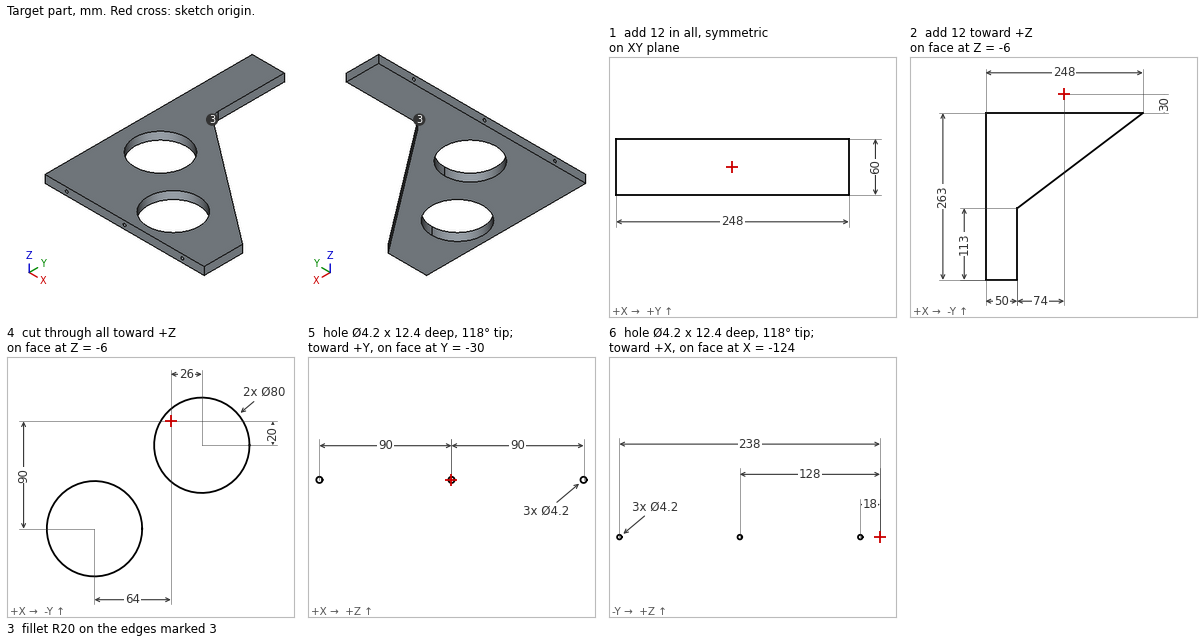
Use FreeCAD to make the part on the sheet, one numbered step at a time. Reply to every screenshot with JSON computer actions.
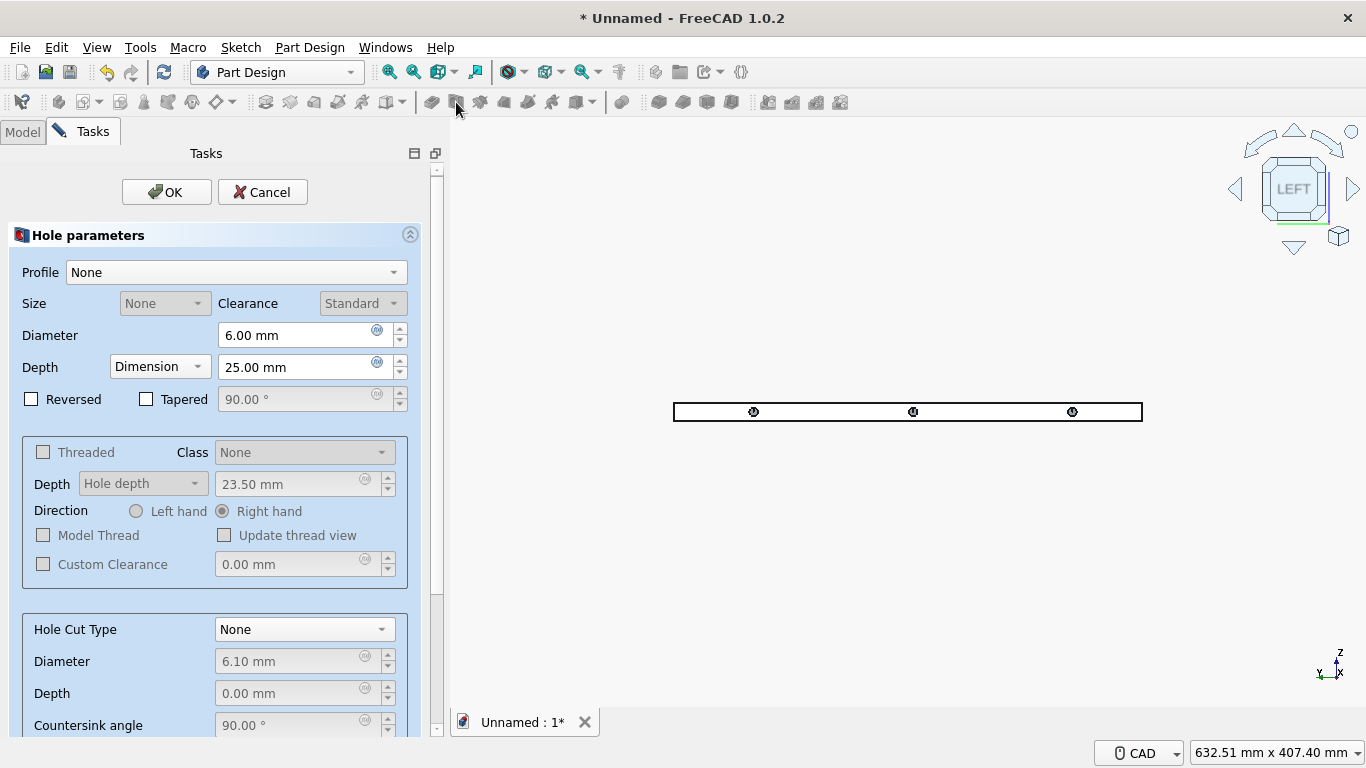
{"action": "triple_click", "coordinate": [305, 335]}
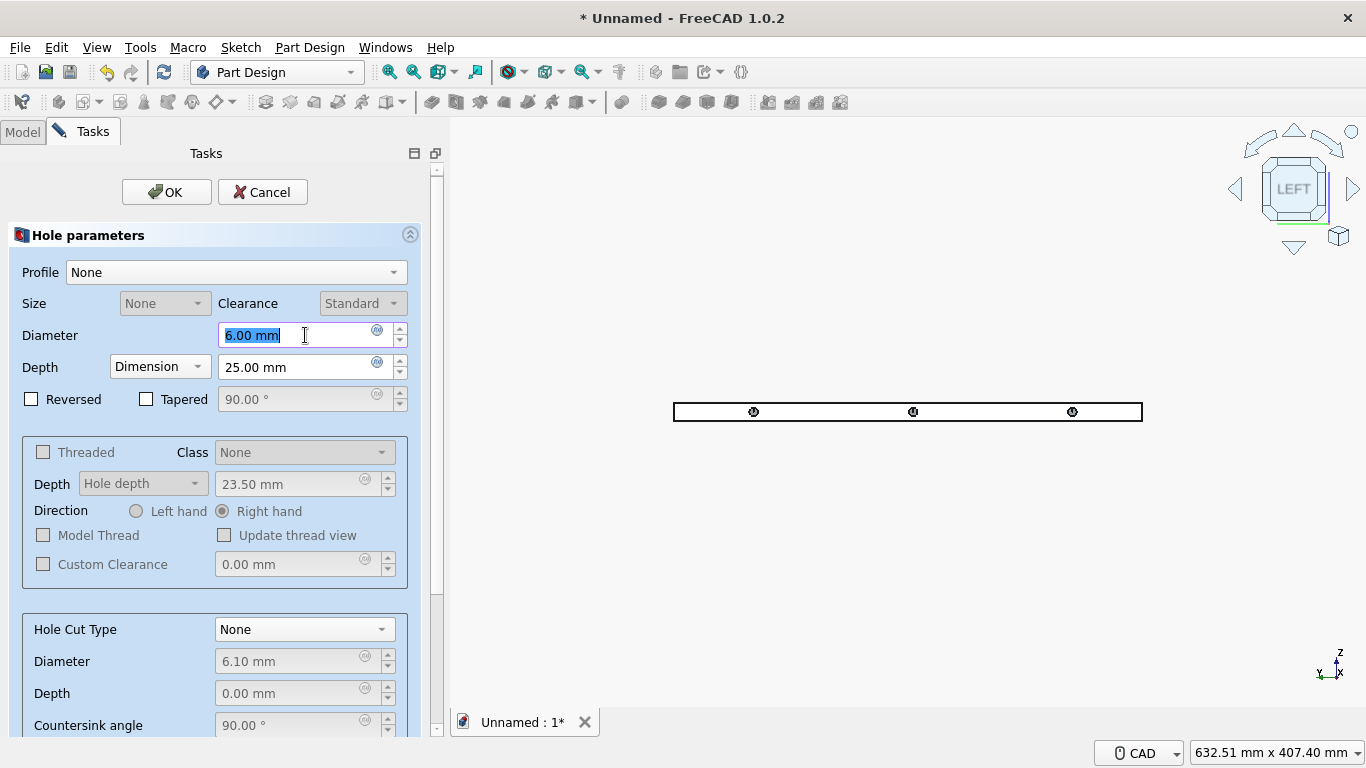
{"action": "type", "text": "4.2"}
{"action": "key", "text": "Tab"}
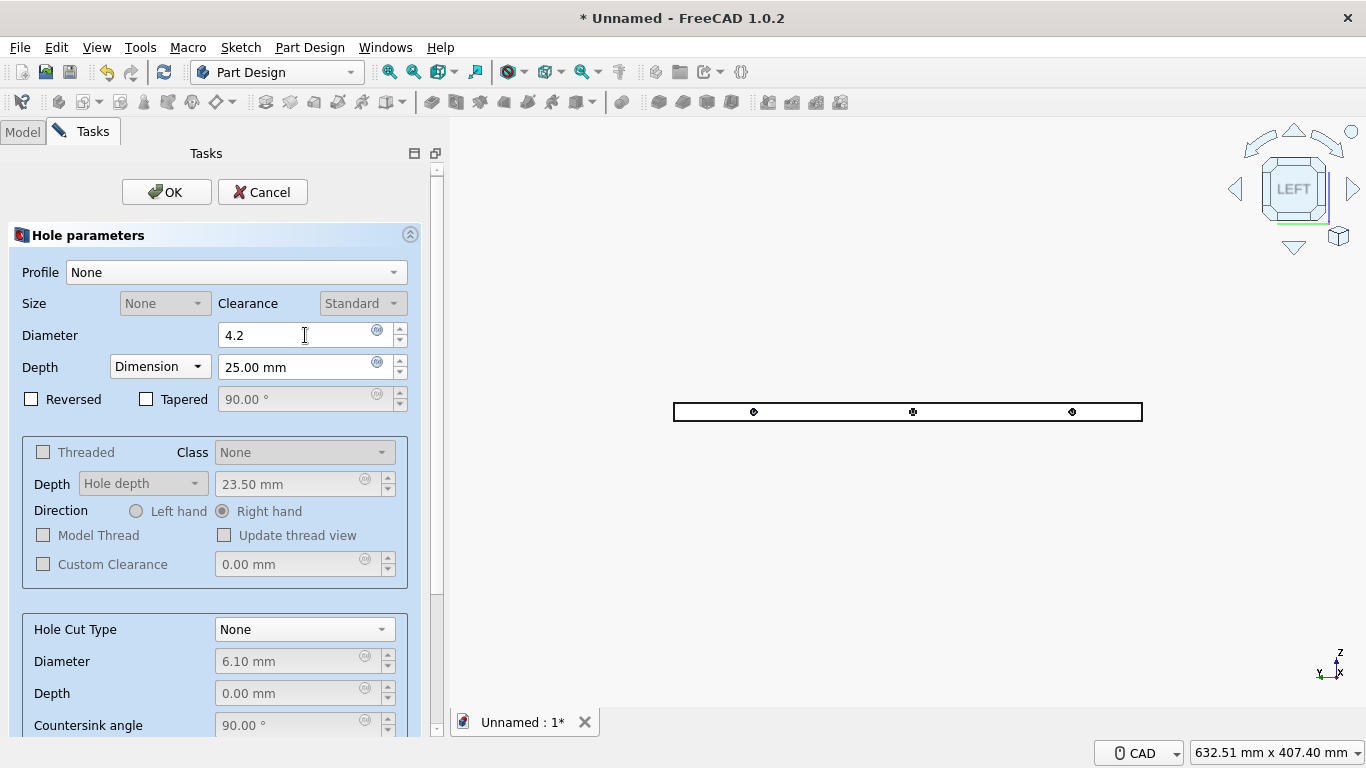
{"action": "triple_click", "coordinate": [305, 367]}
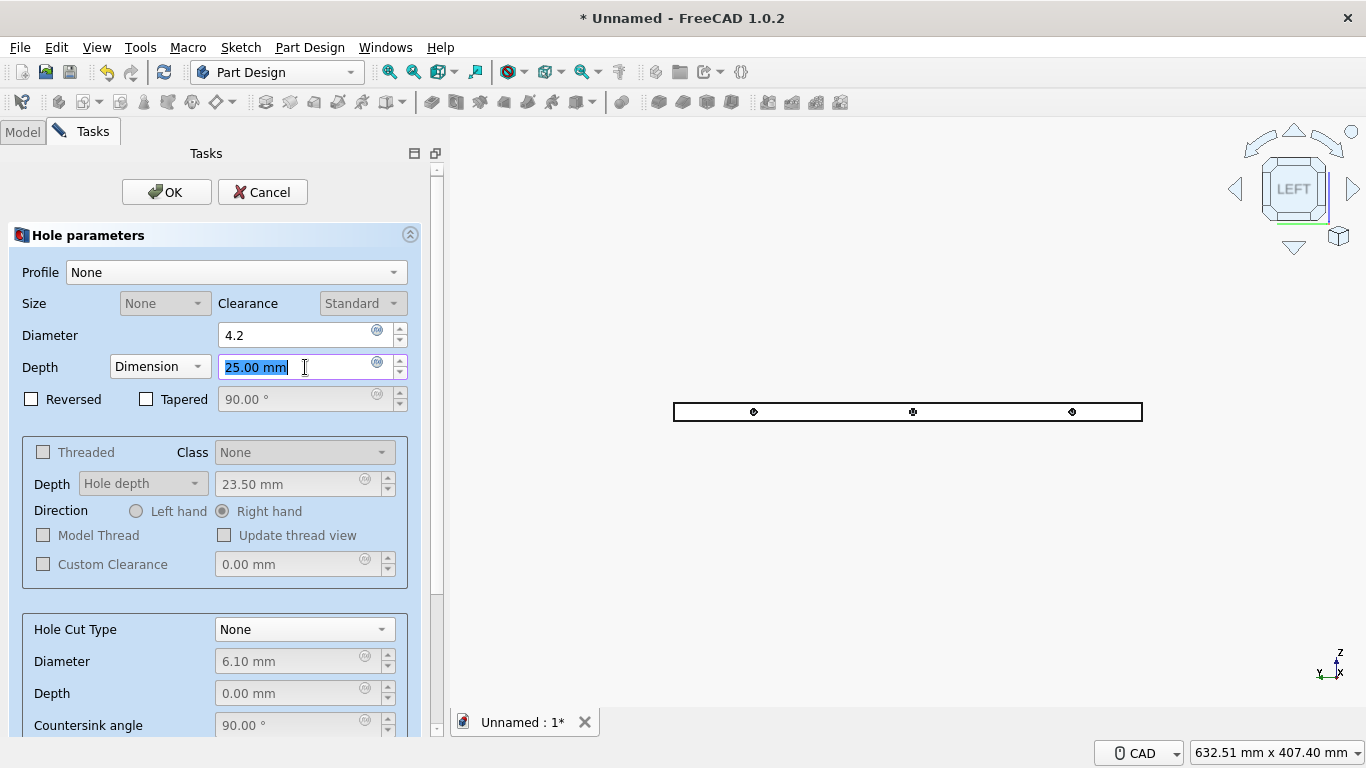
{"action": "type", "text": "12.4"}
{"action": "key", "text": "Tab"}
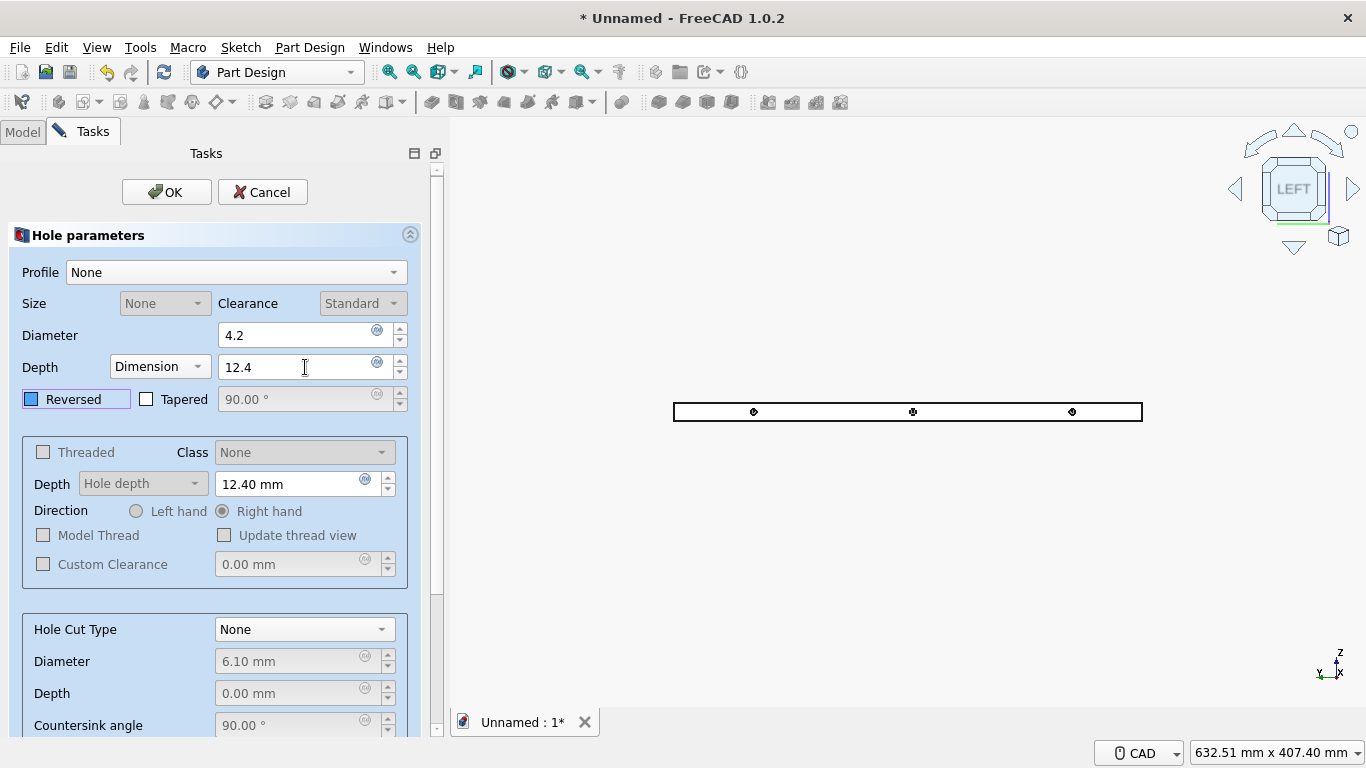
{"action": "left_click", "coordinate": [167, 192]}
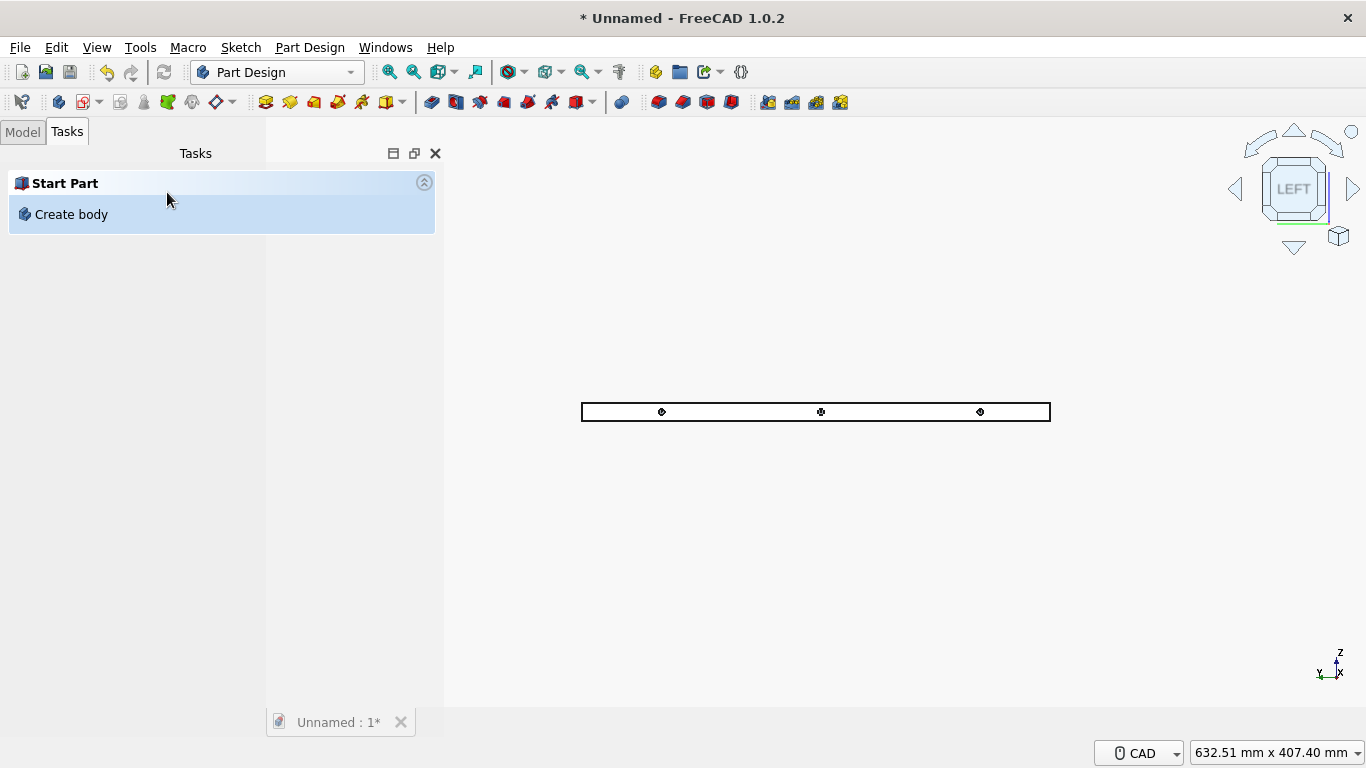
{"action": "key", "text": "0"}